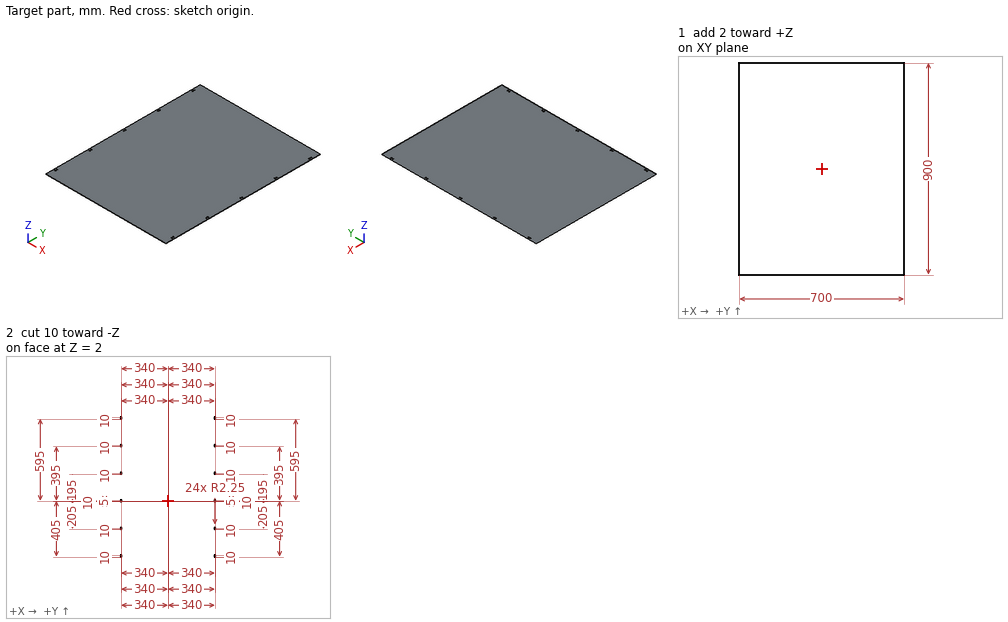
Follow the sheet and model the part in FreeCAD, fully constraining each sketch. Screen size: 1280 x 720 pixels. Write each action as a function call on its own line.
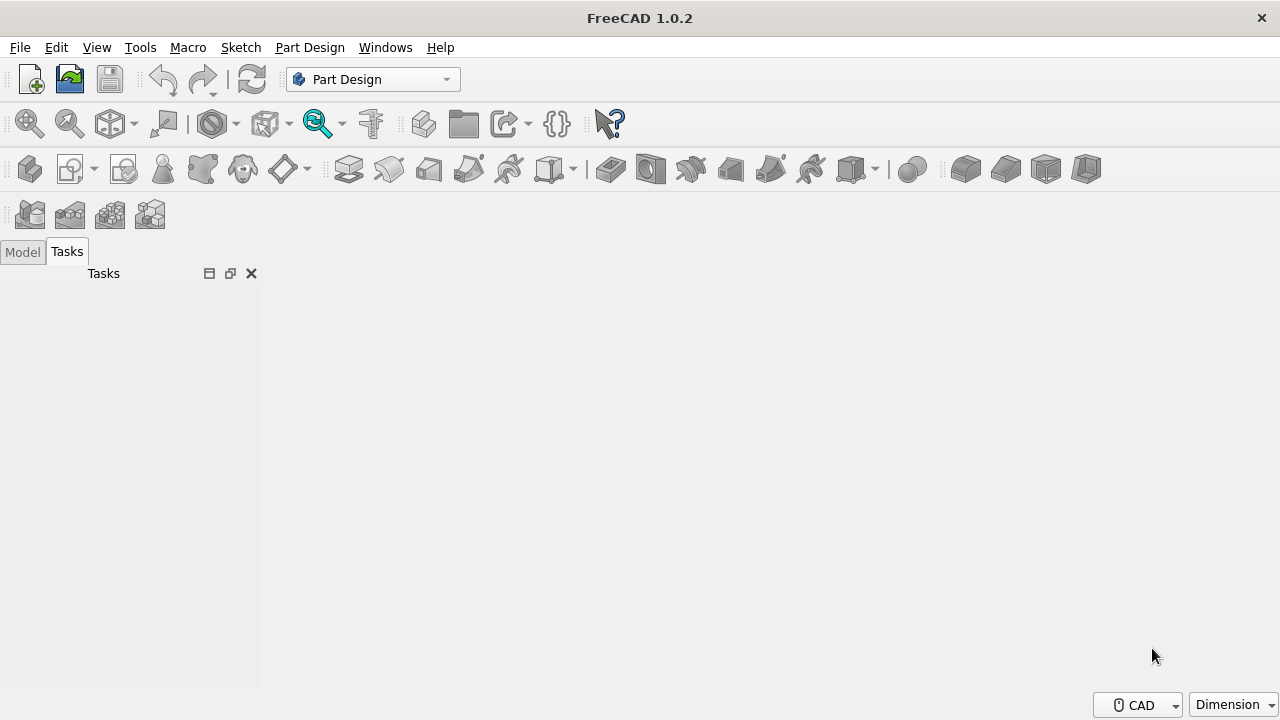
click(30, 80)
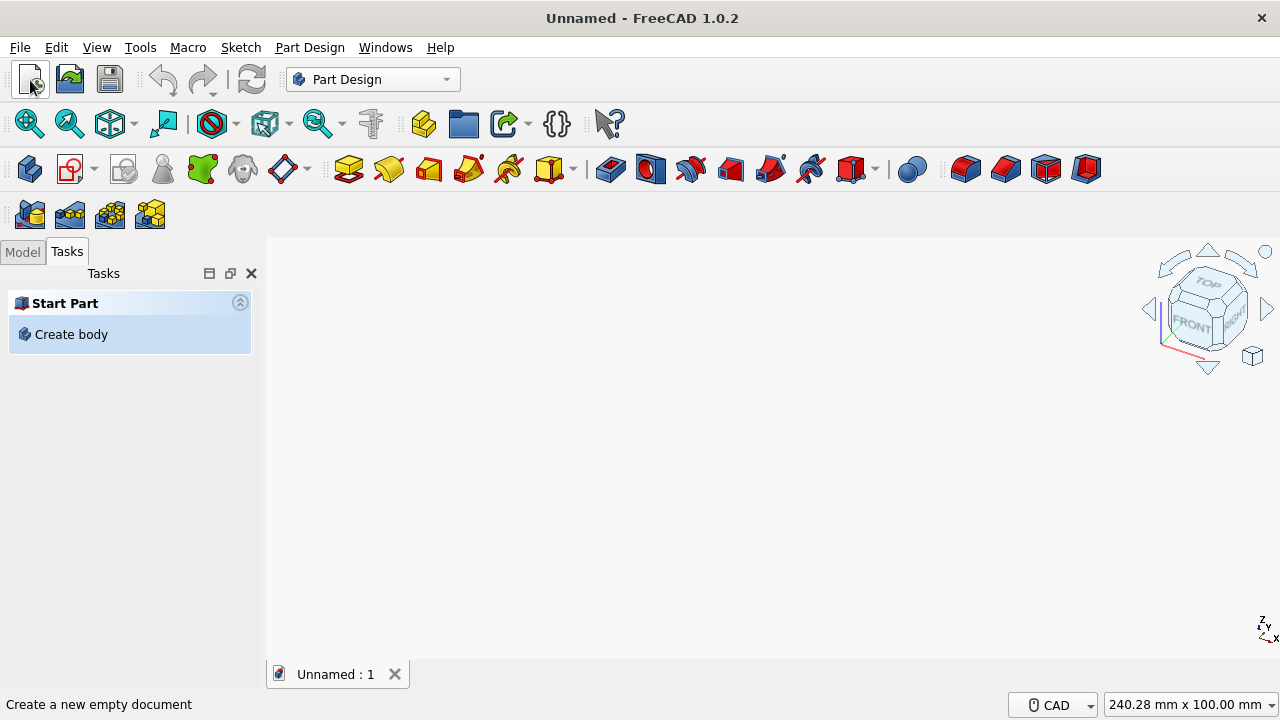
click(70, 170)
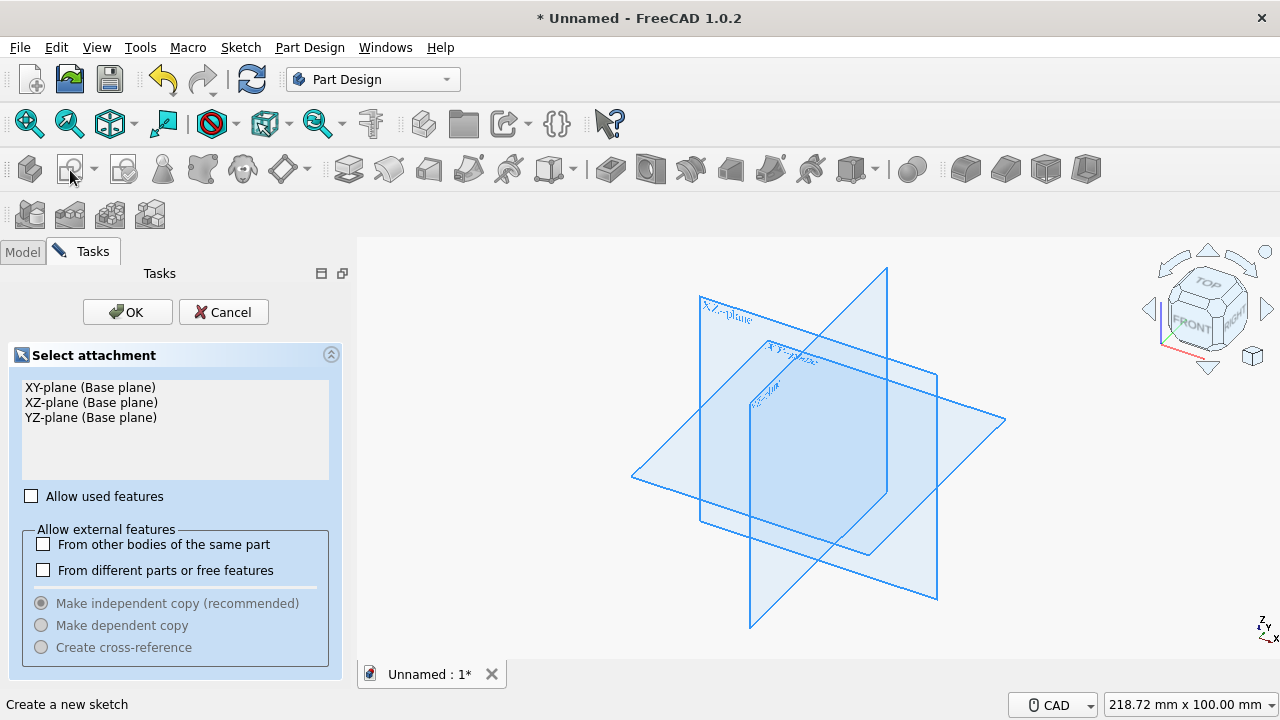
click(82, 388)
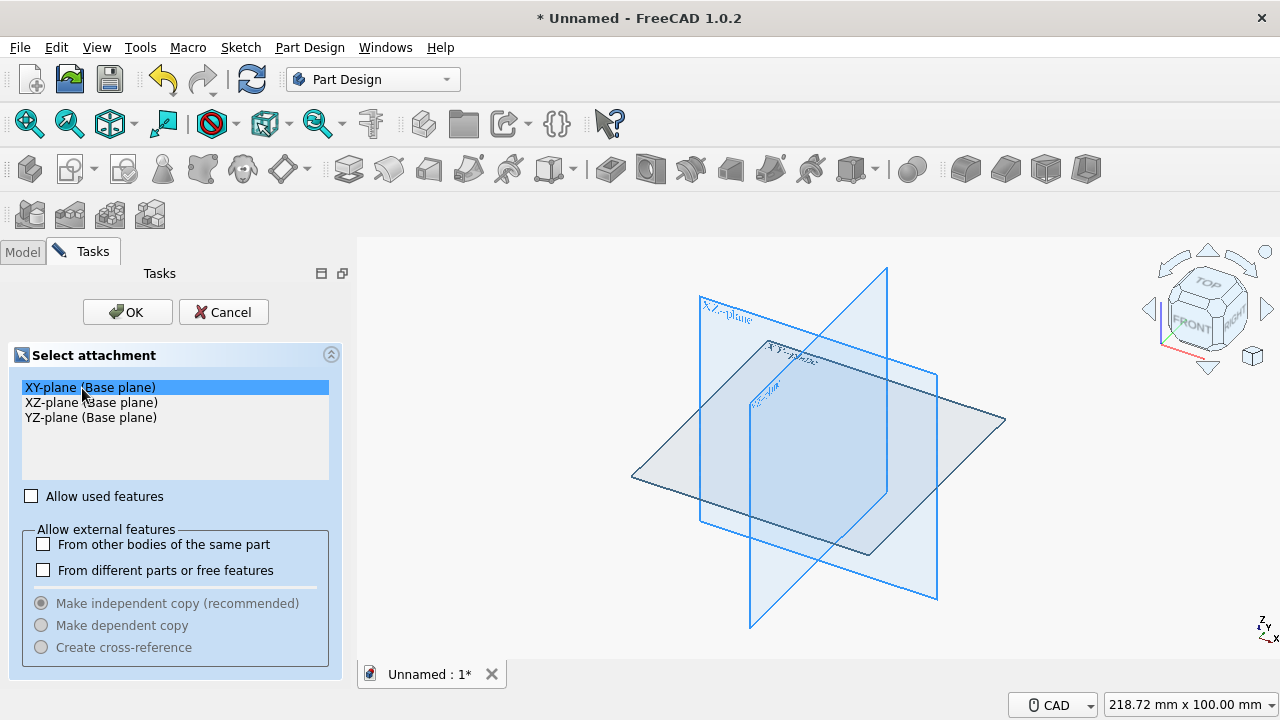
click(128, 312)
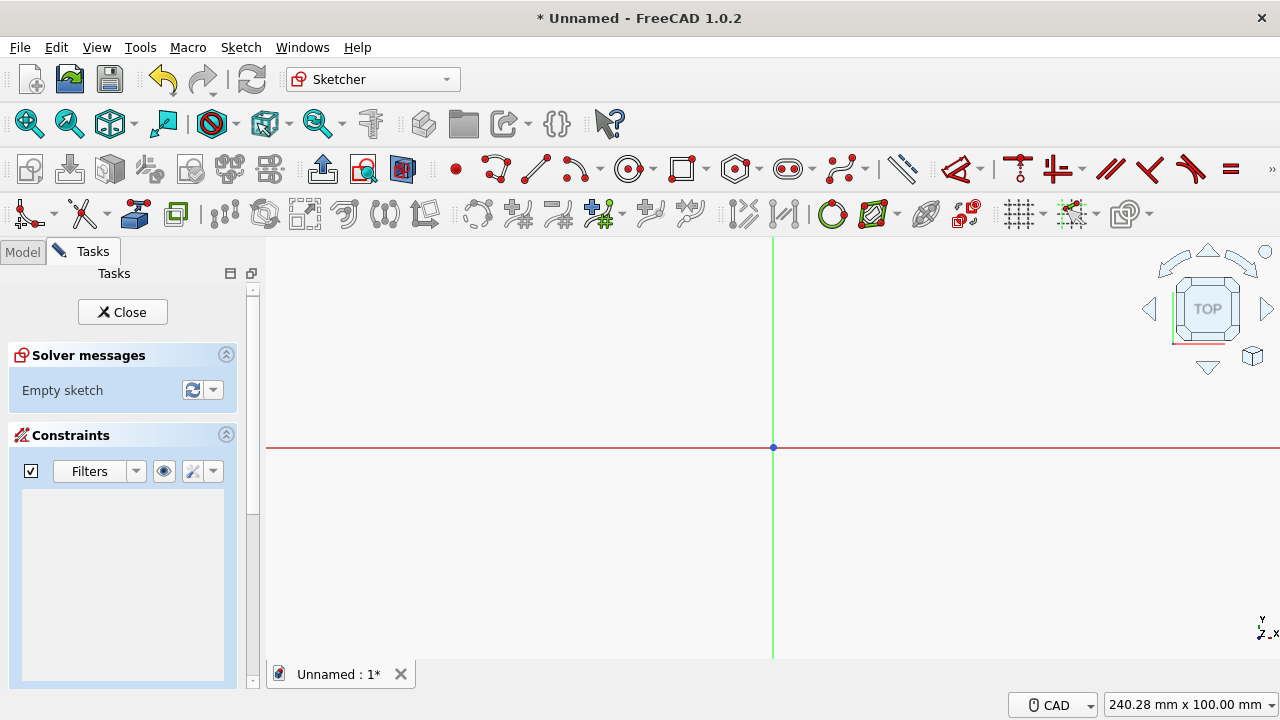
scroll(699, 448, down, 13)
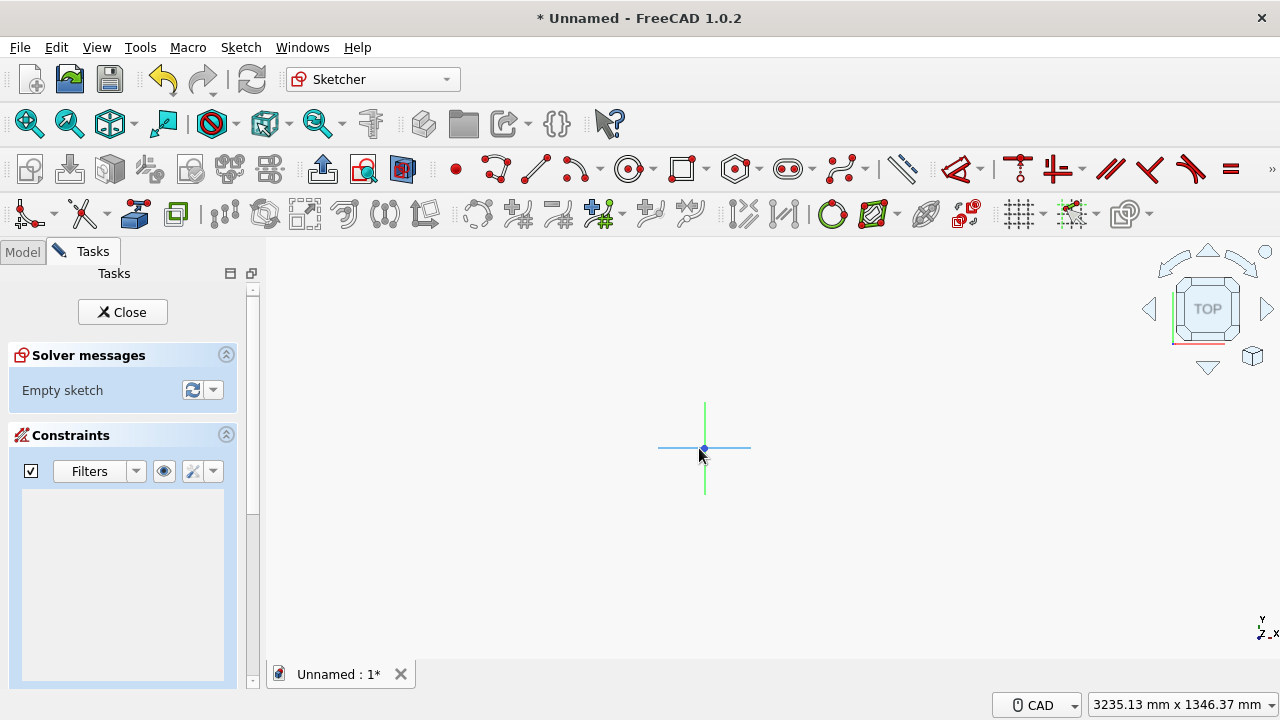
key(g)
key(v)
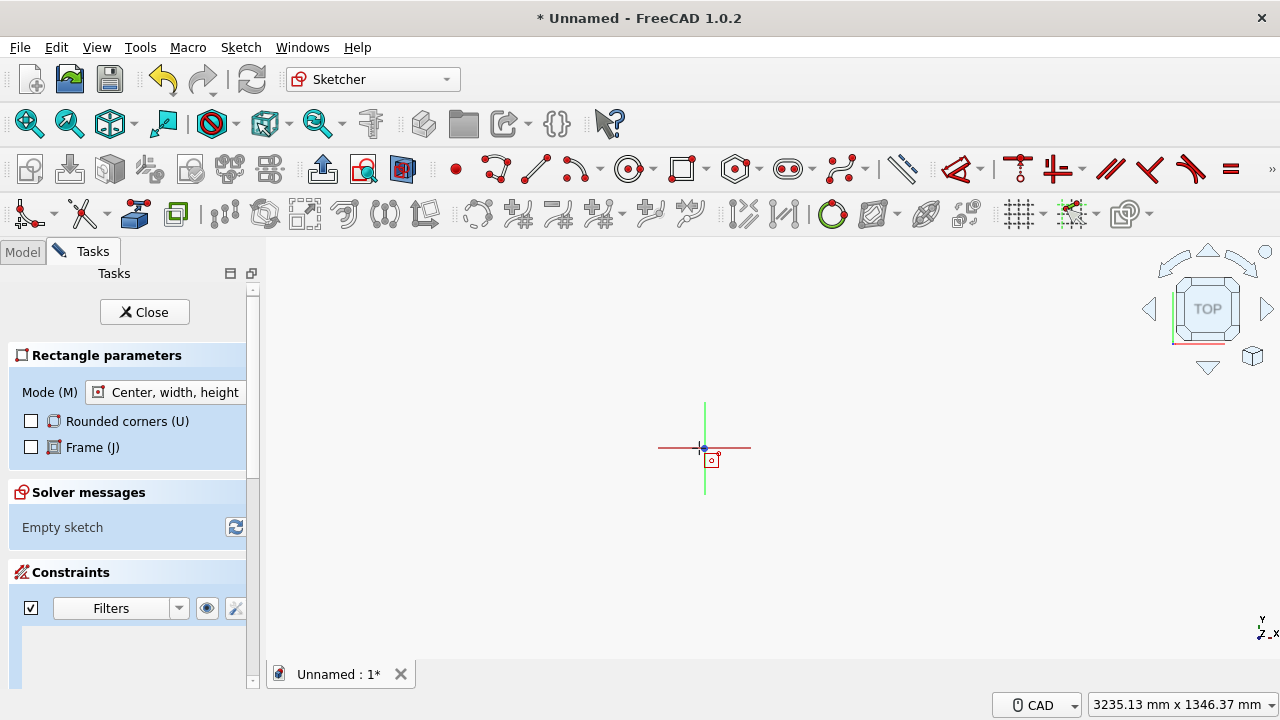
click(705, 448)
move(815, 307)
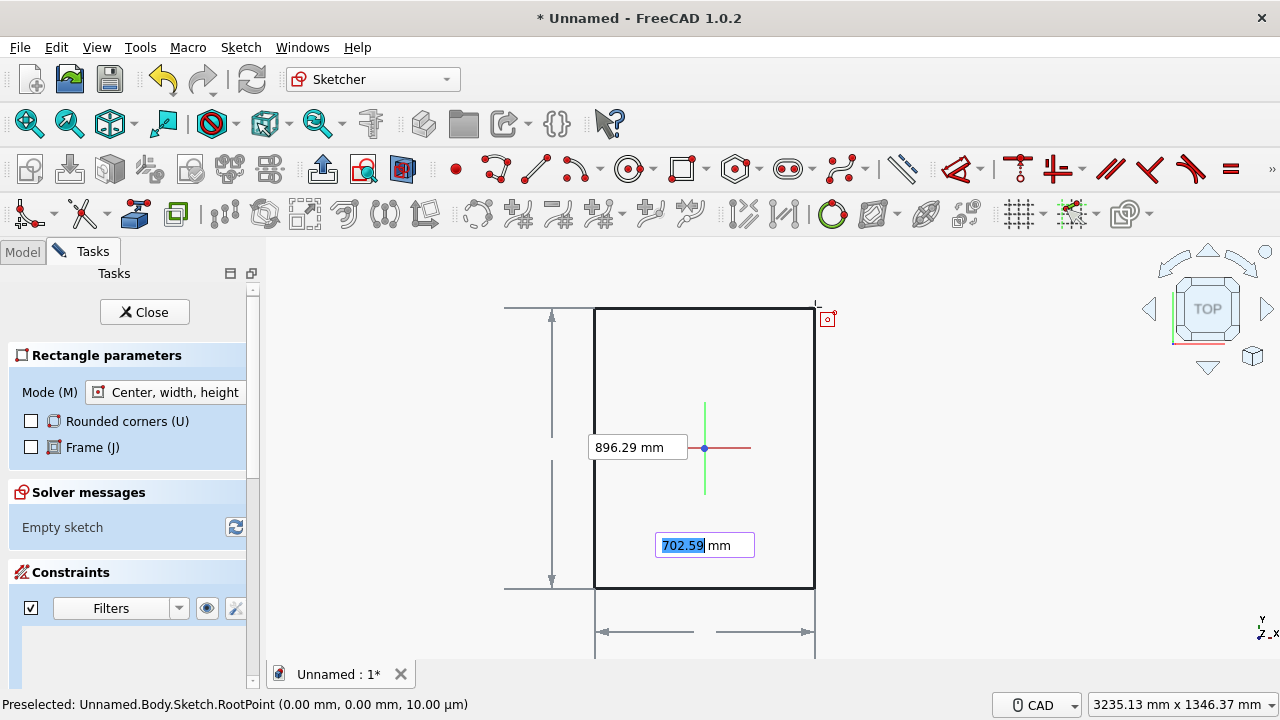
text(700)
key(Tab)
text(900)
key(Return)
key(Escape)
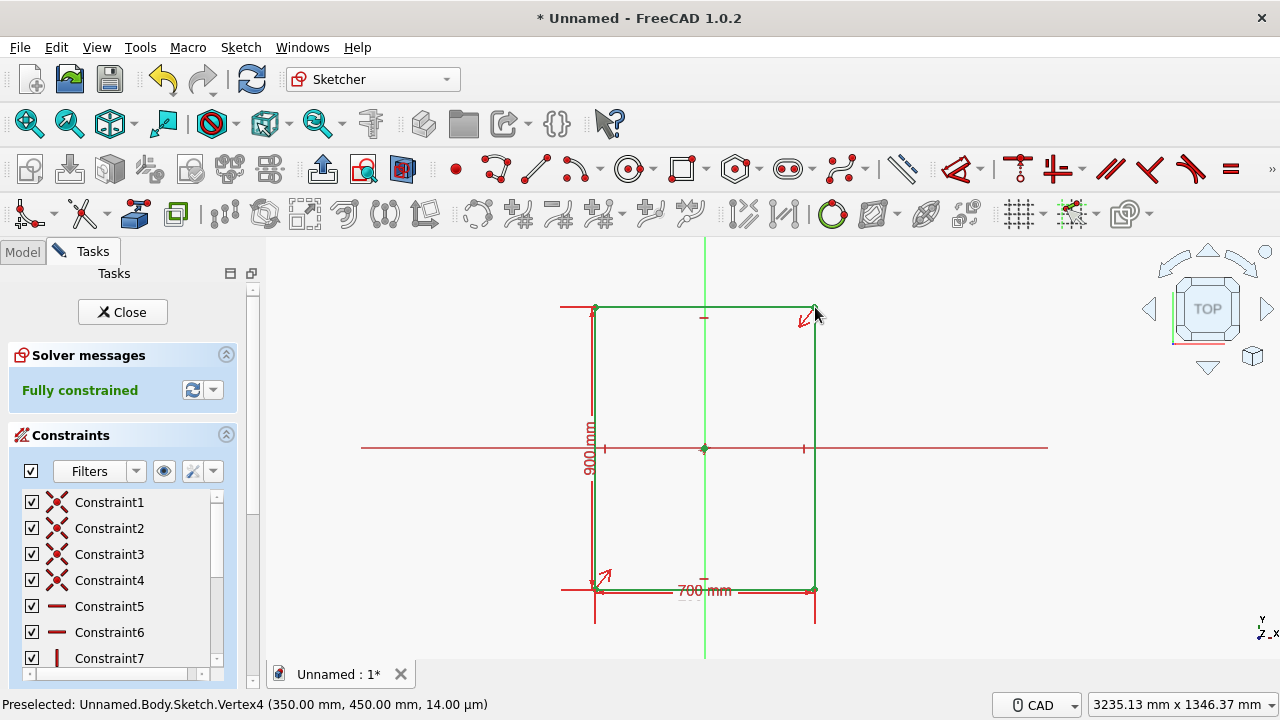
click(123, 312)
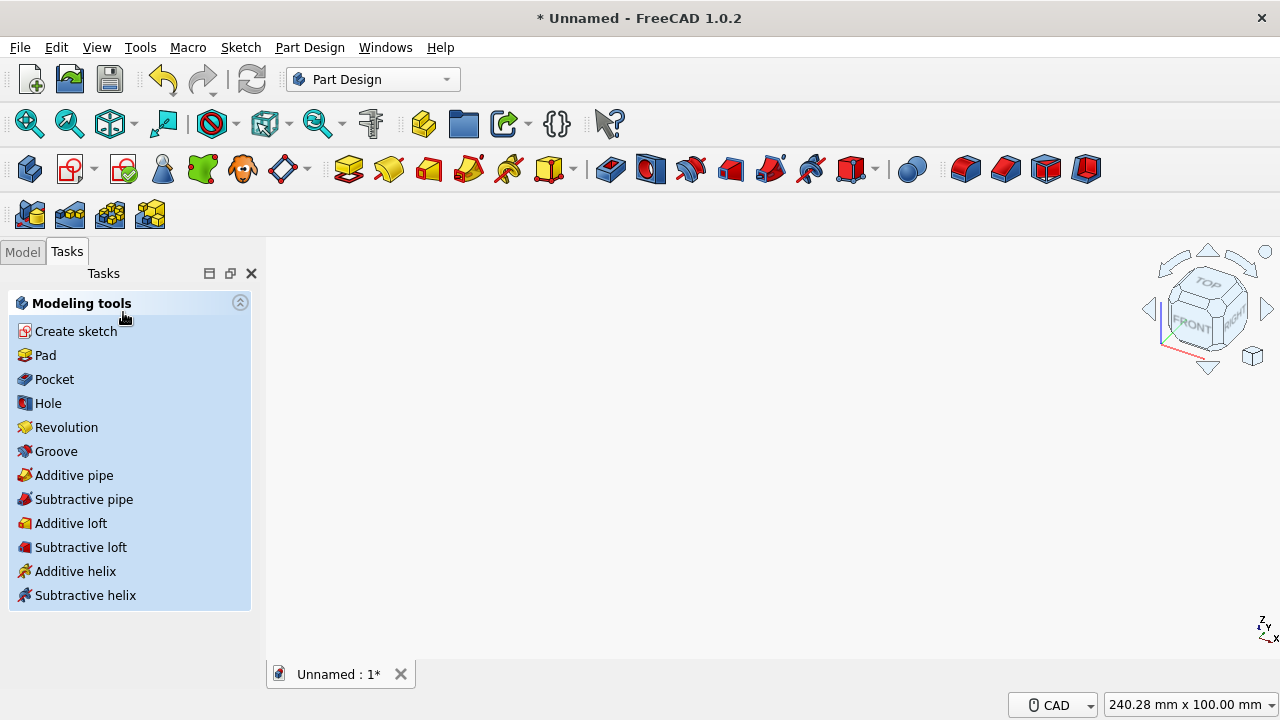
click(350, 170)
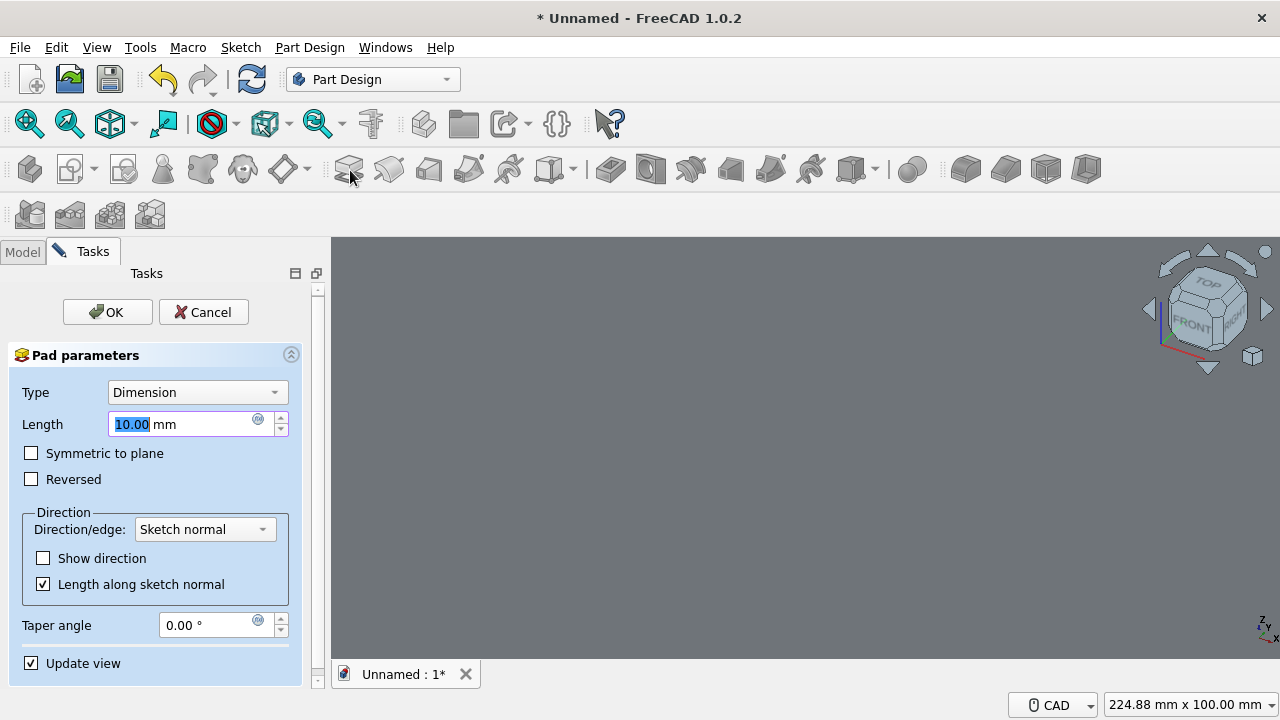
text(2)
key(Tab)